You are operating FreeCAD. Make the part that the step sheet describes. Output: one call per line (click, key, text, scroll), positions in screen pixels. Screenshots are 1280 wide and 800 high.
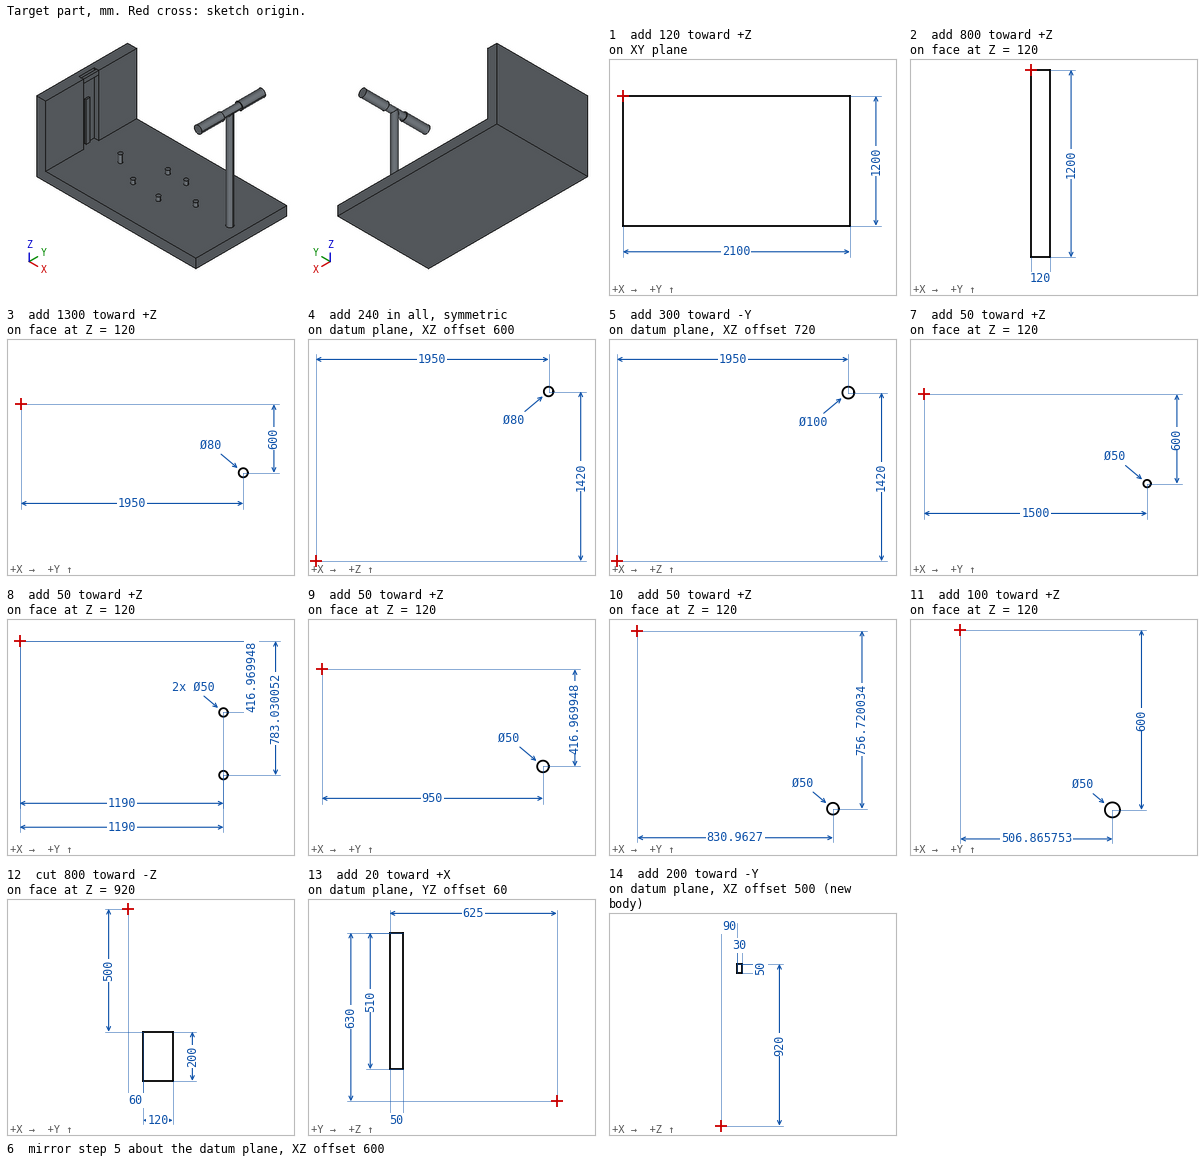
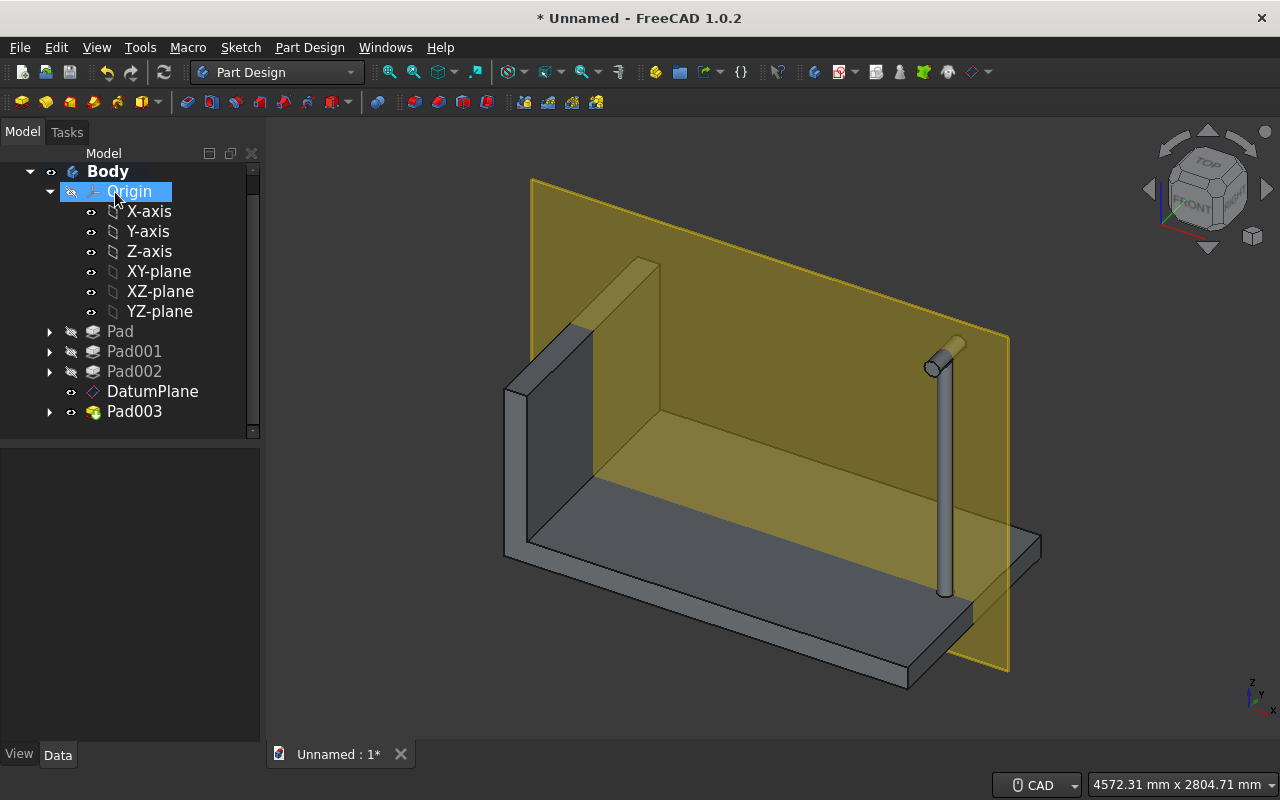
click(116, 392)
key(space)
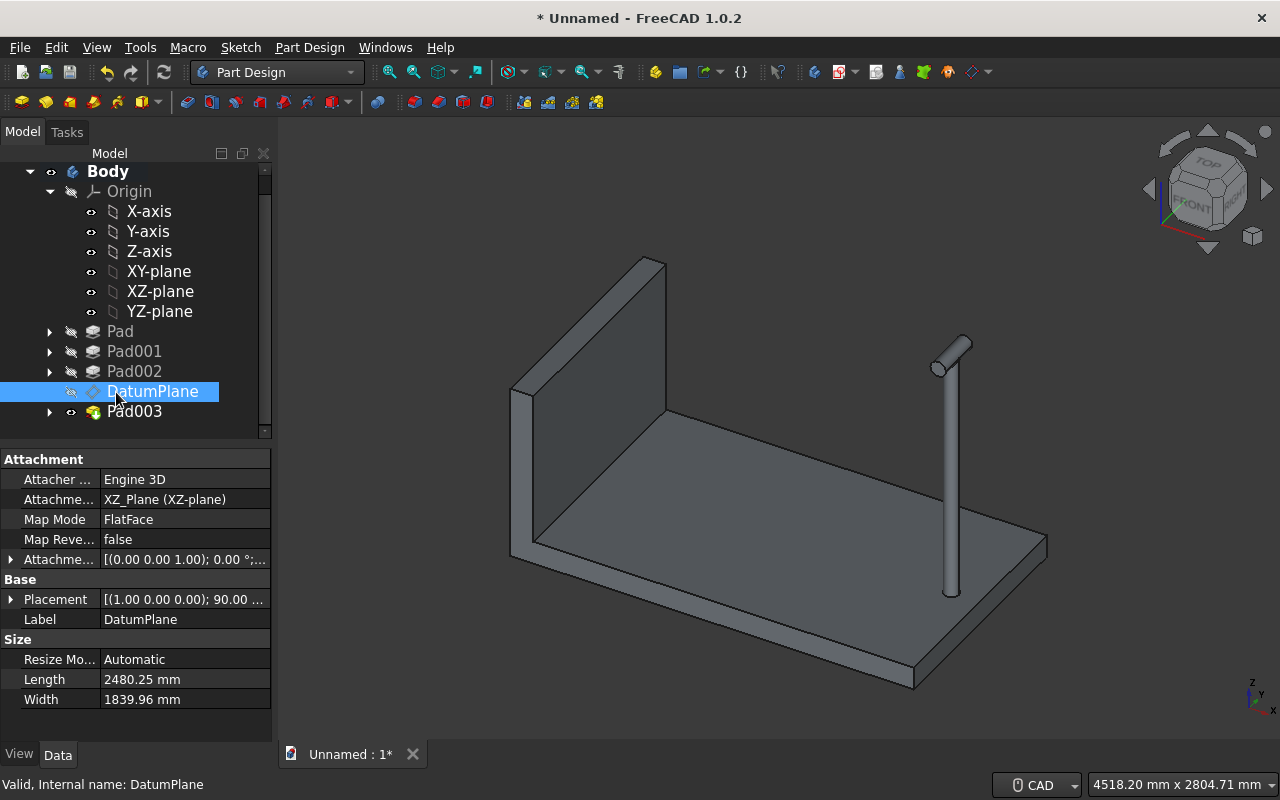
key(0)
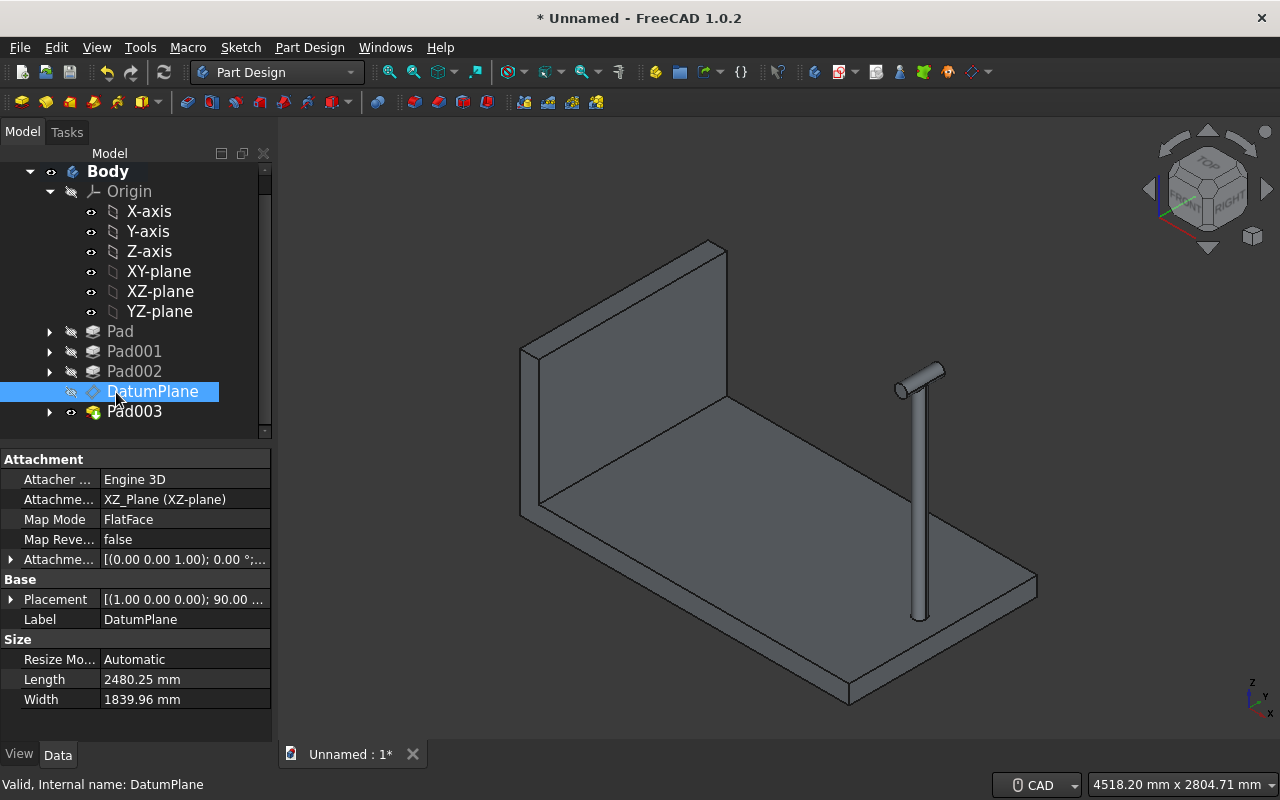
key(1)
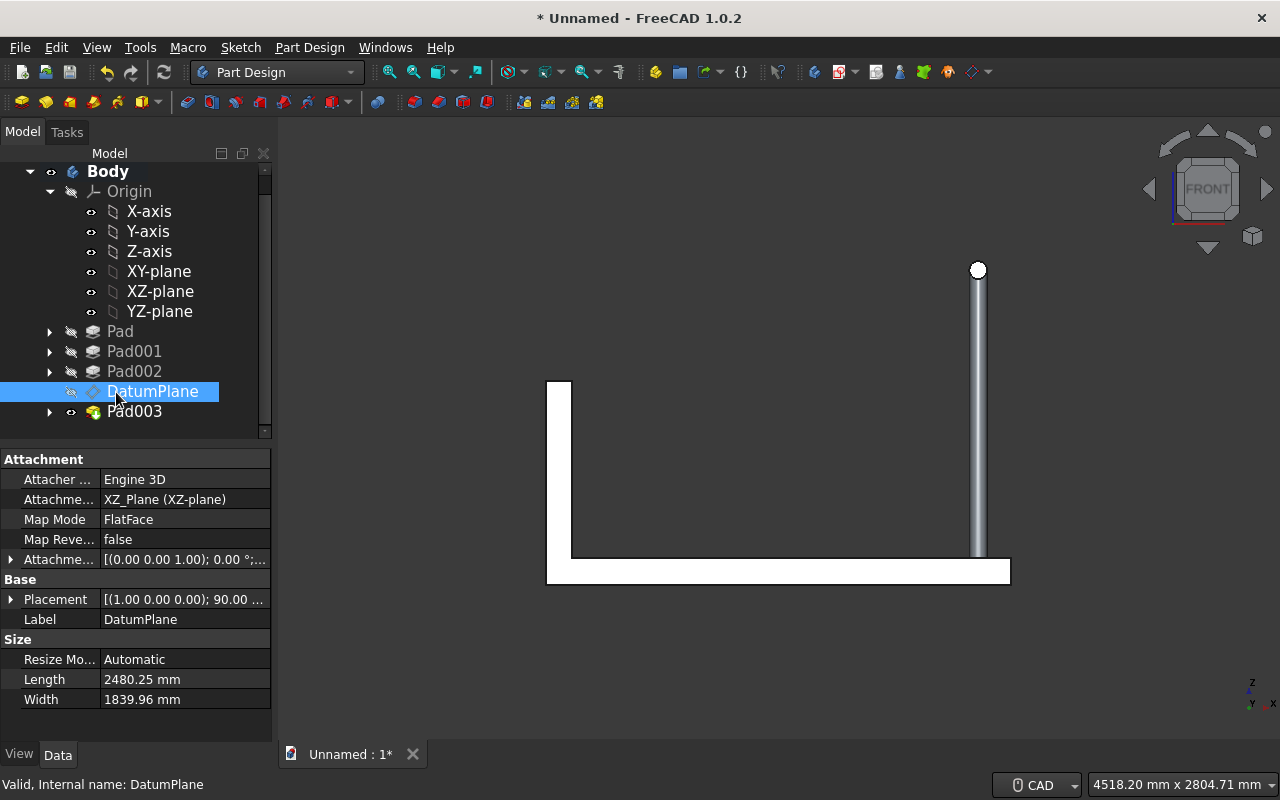
key(2)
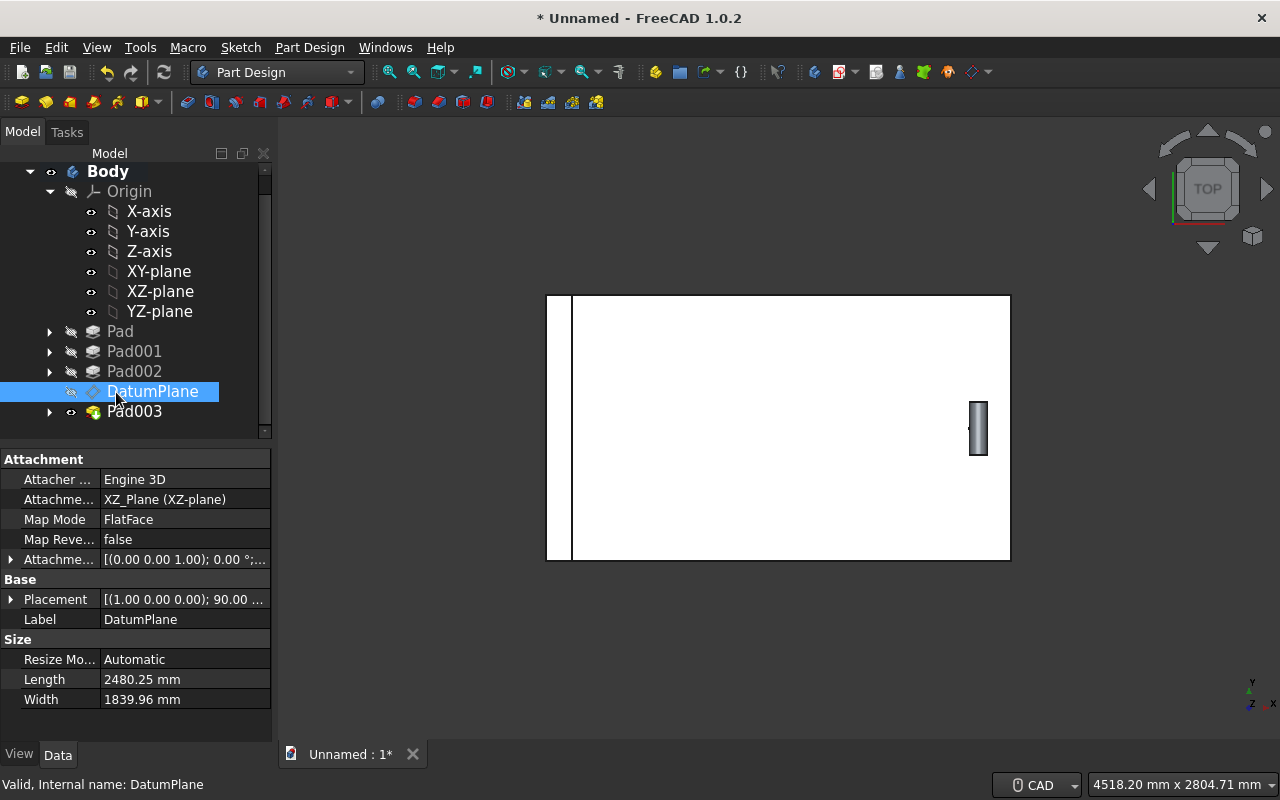
click(136, 292)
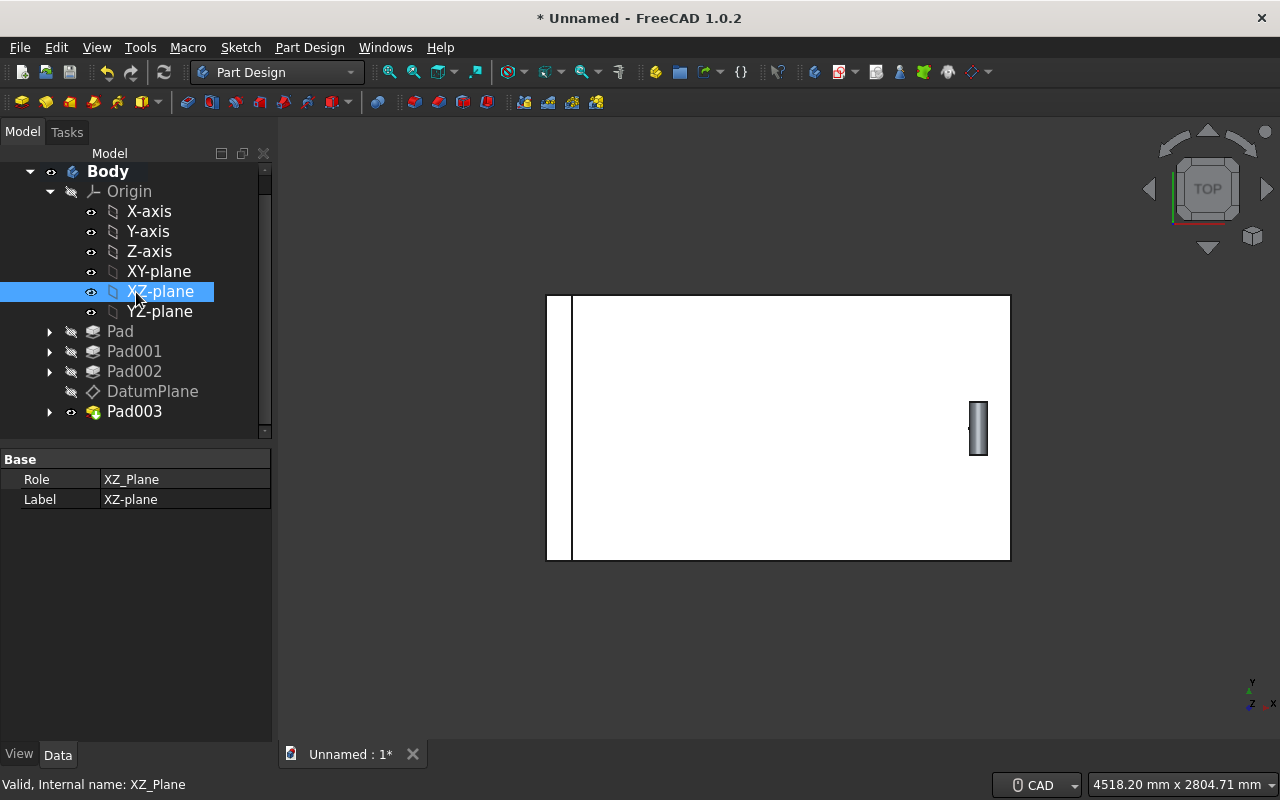
click(972, 72)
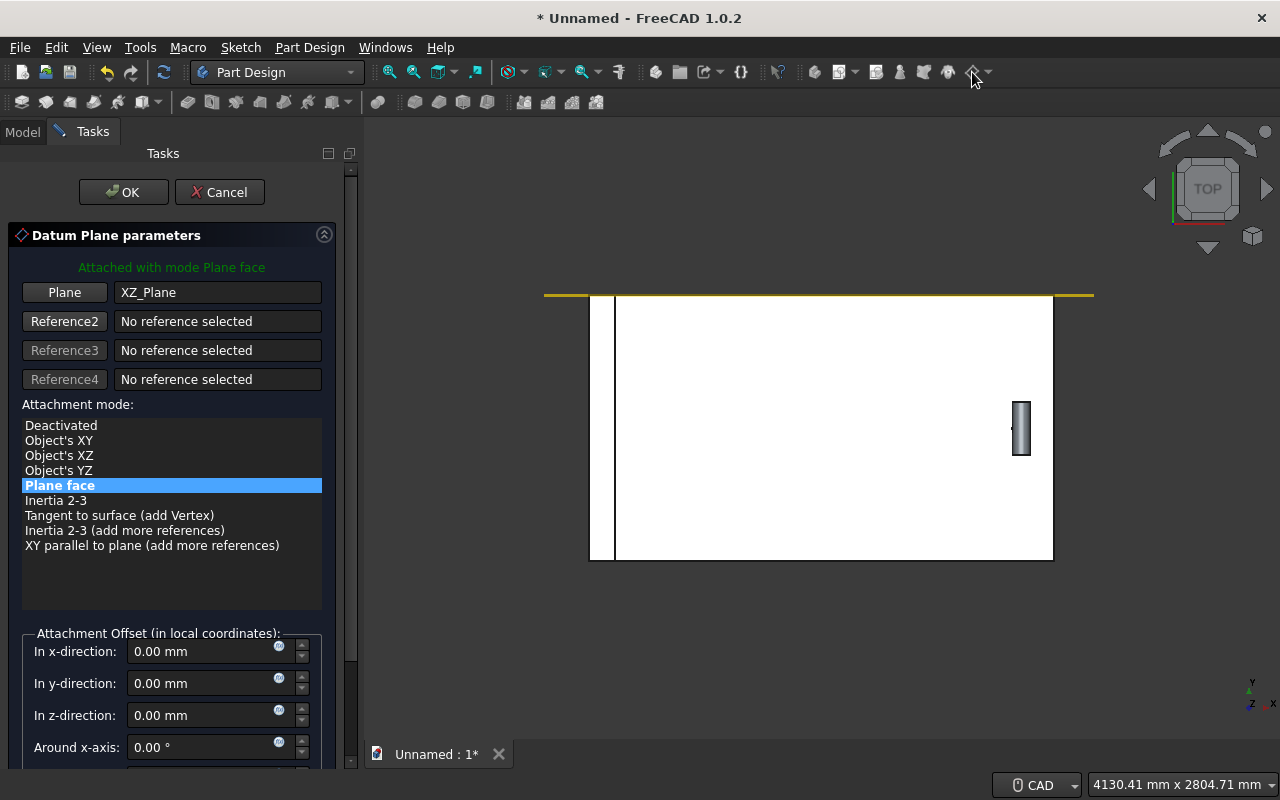
triple_click(210, 715)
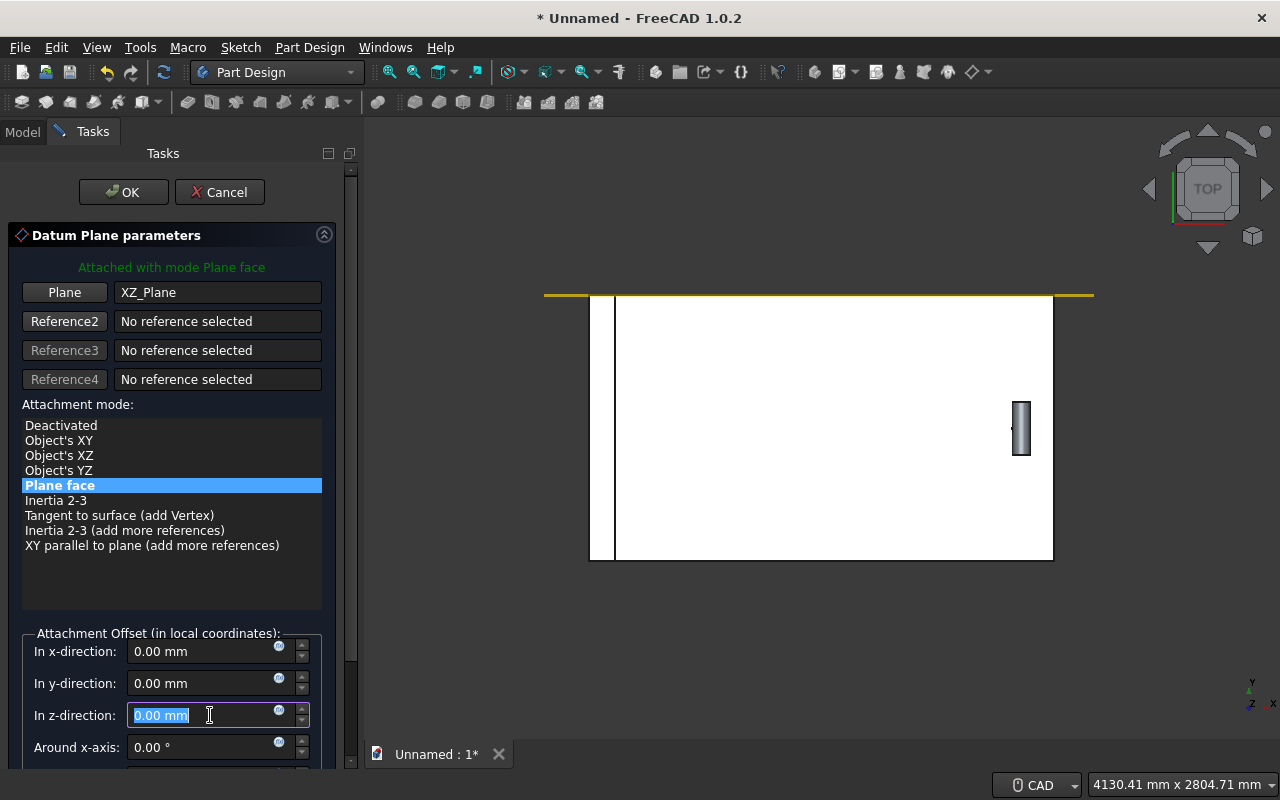
text(720)
key(Tab)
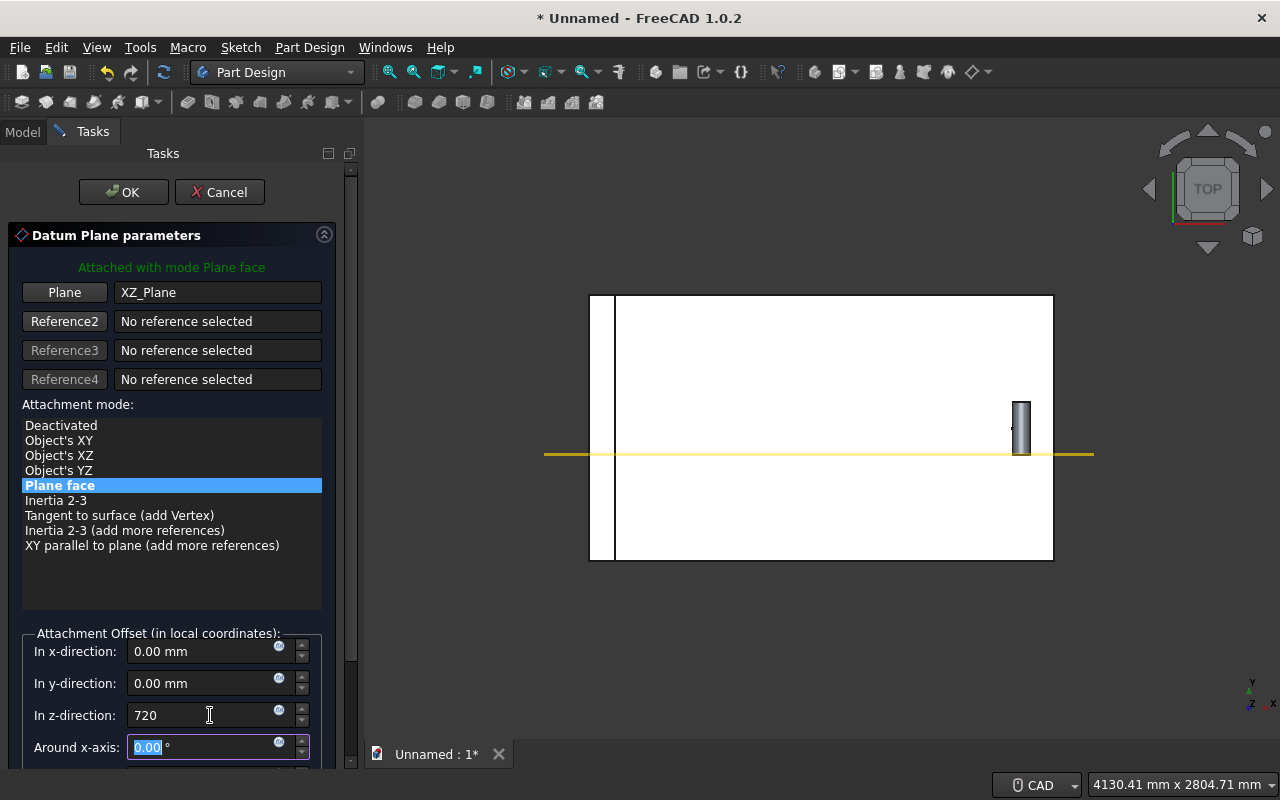
click(124, 192)